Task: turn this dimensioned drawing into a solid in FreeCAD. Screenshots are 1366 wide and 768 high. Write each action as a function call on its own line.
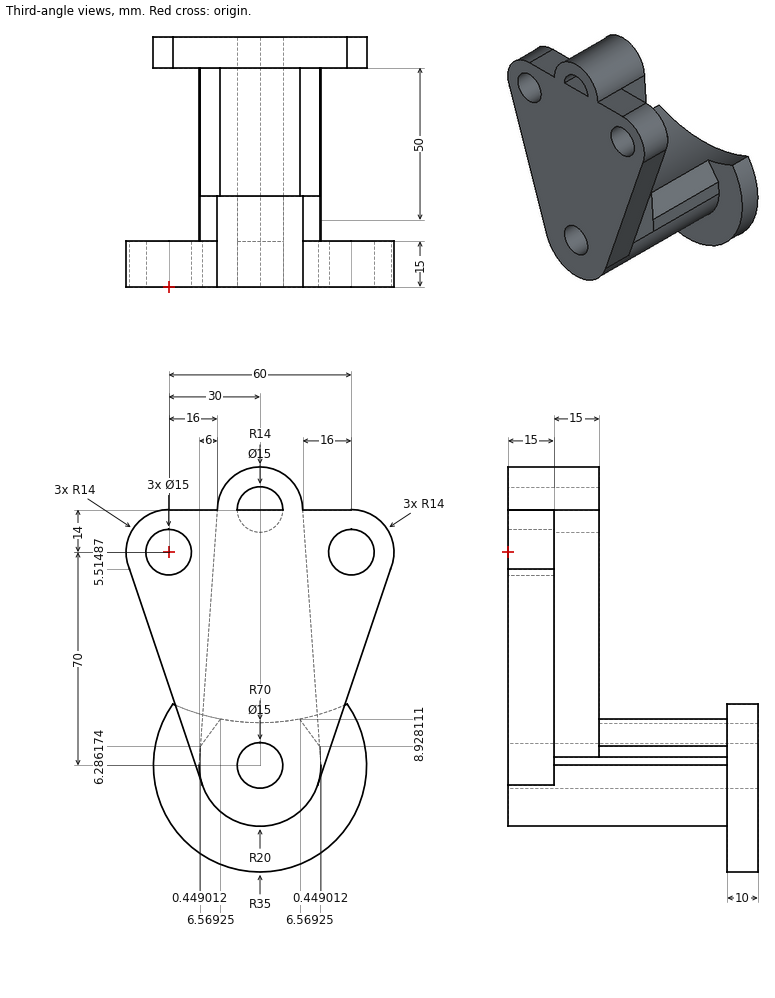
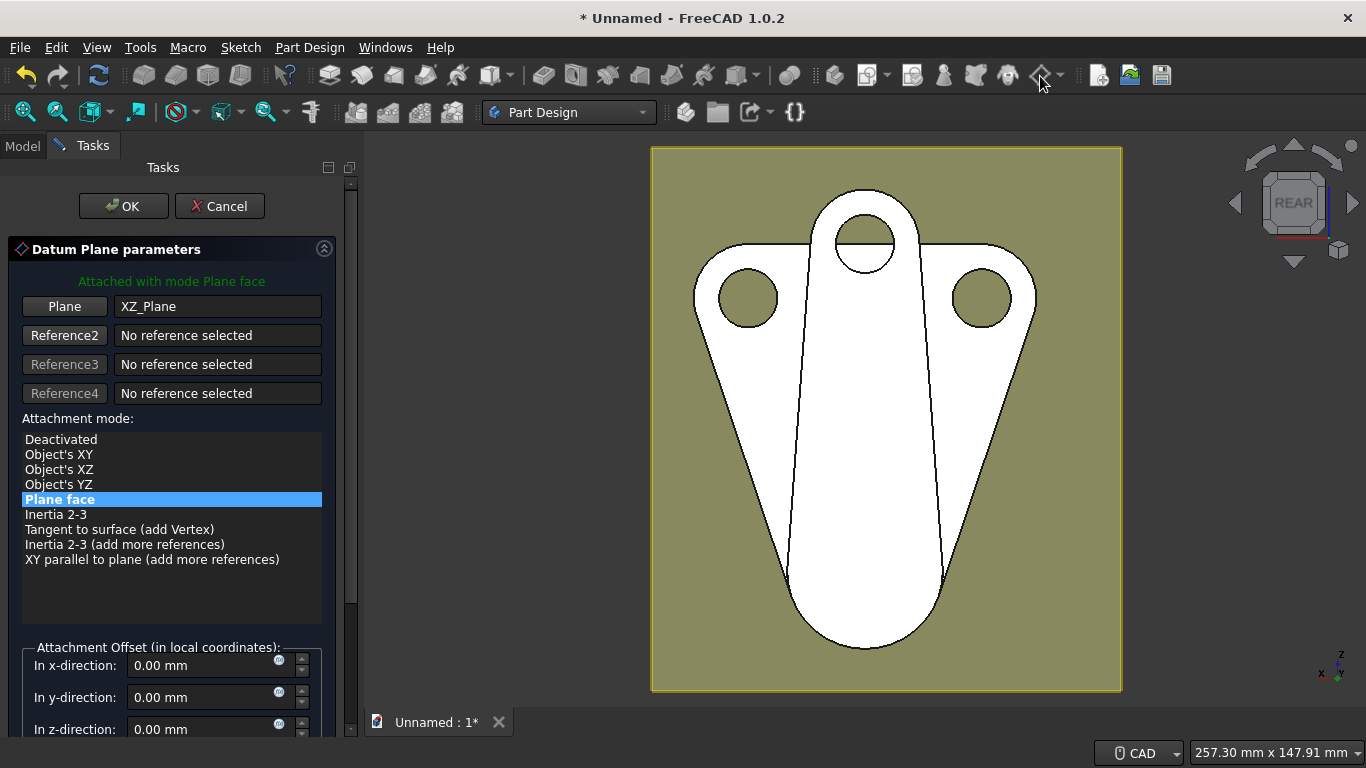
scroll(351, 456, down, 2)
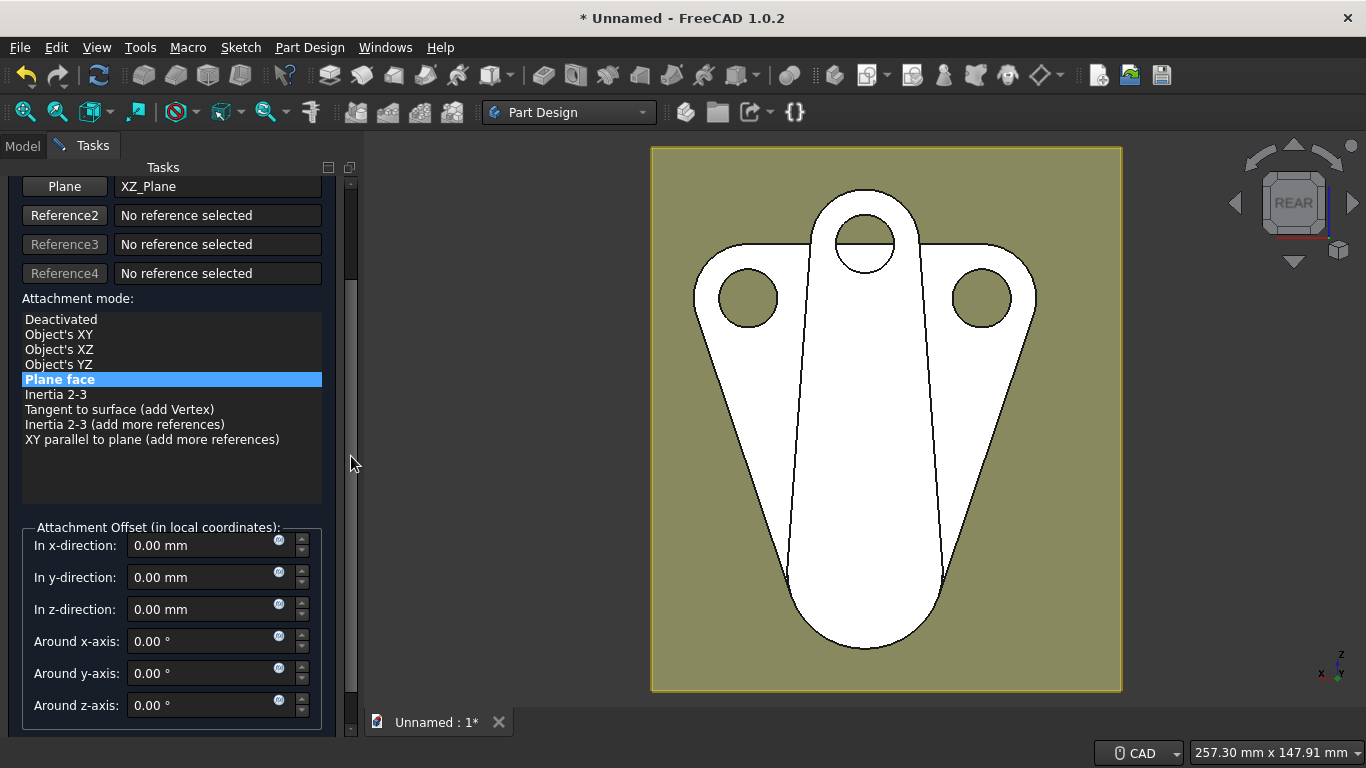
triple_click(210, 609)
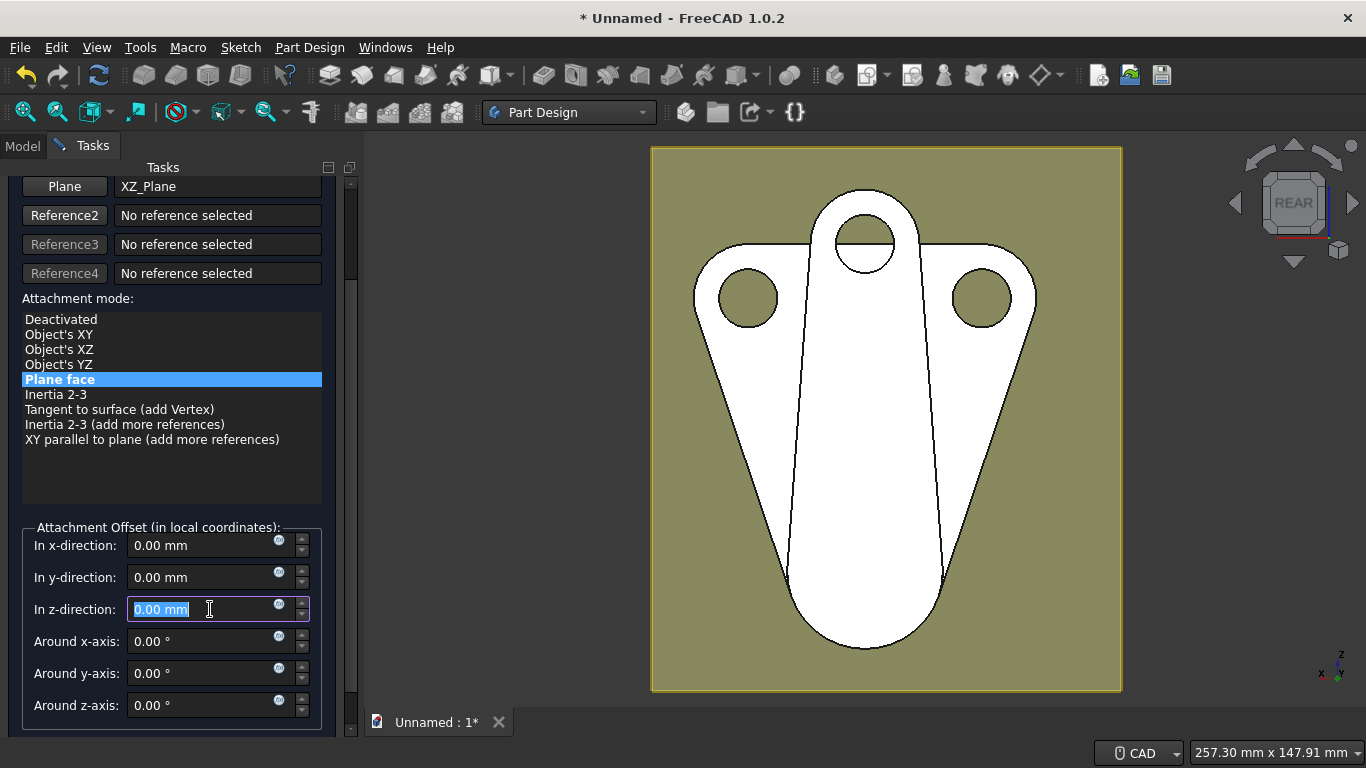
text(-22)
key(Tab)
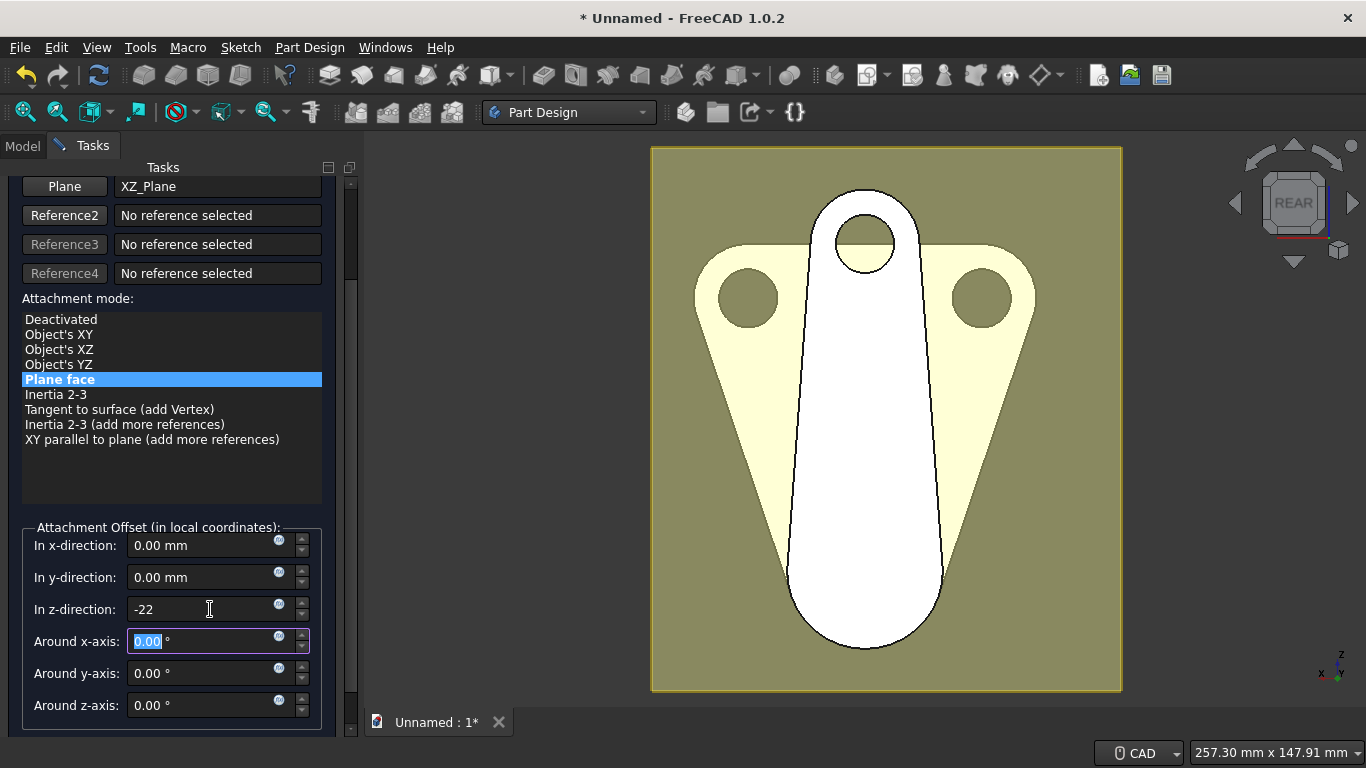
scroll(351, 456, up, 3)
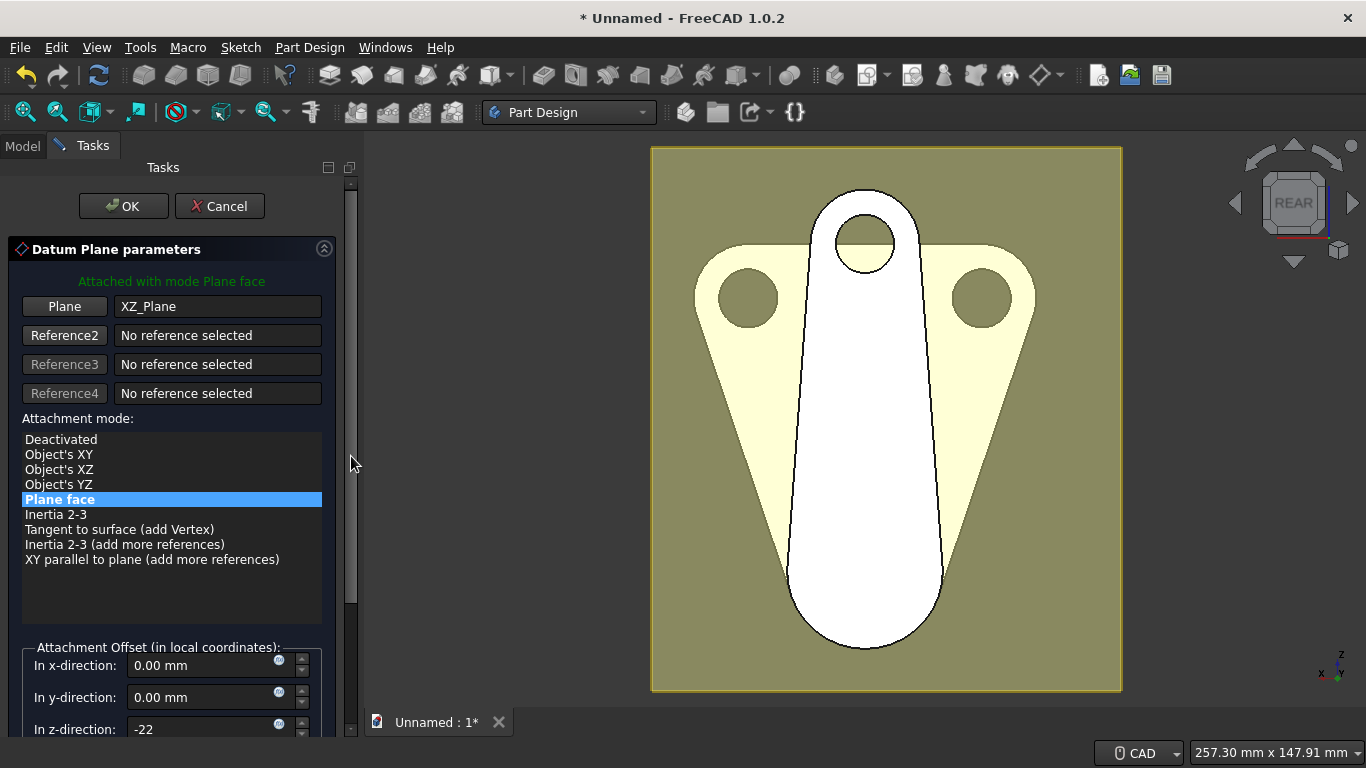
click(124, 206)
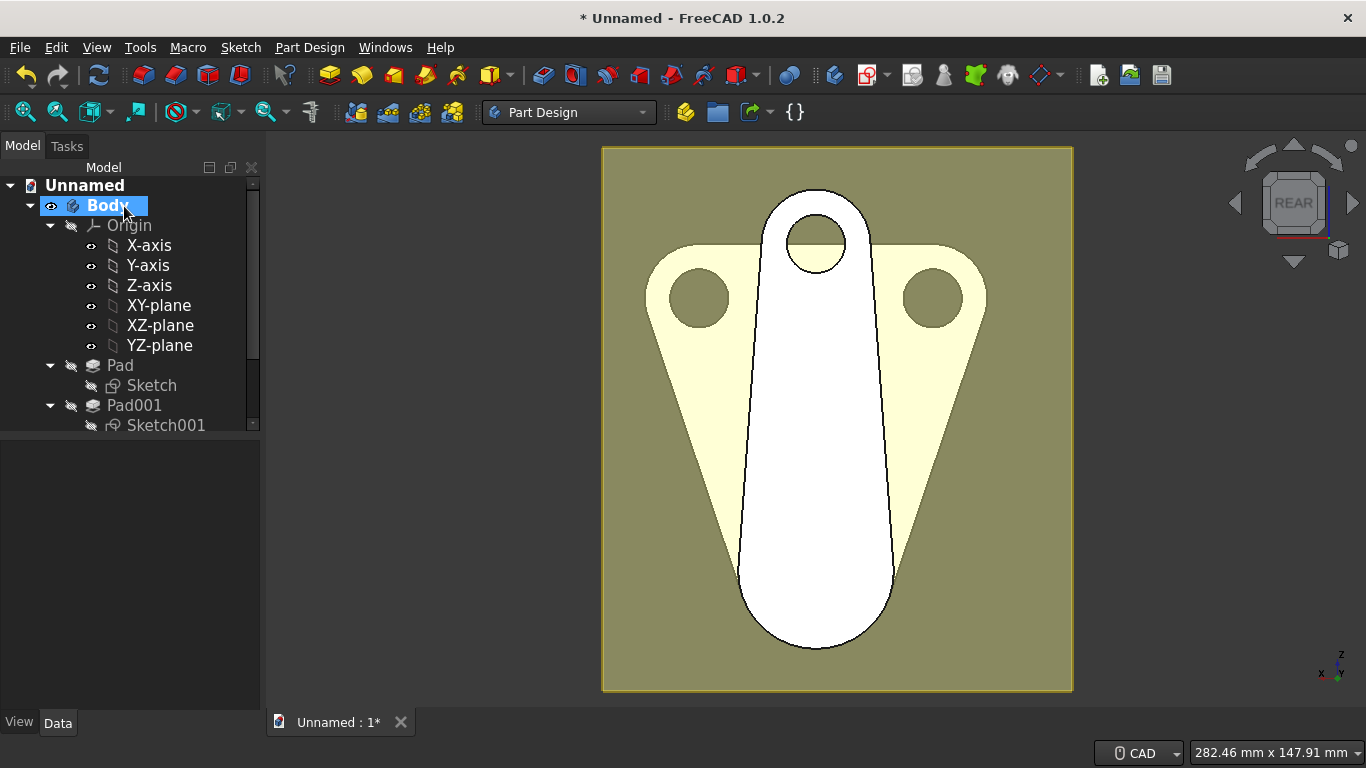
scroll(100, 301, down, 3)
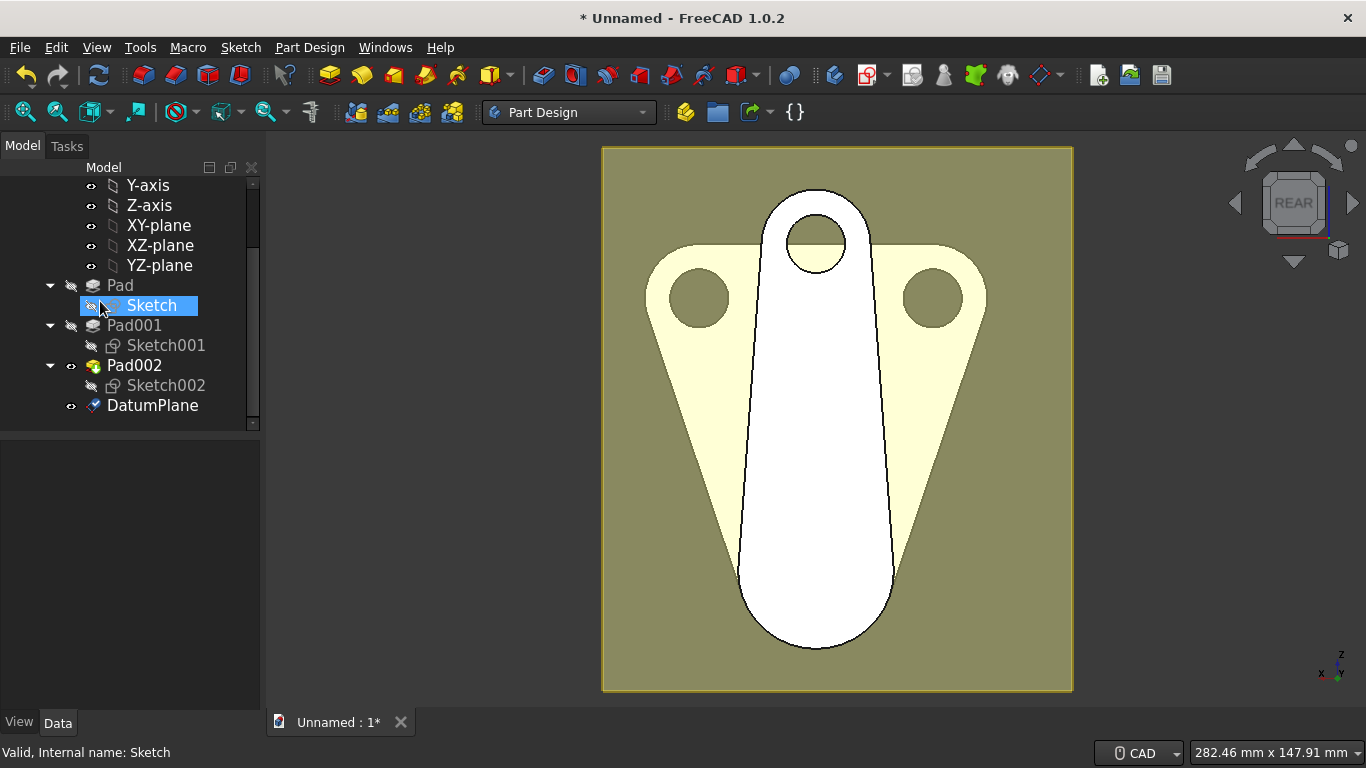
click(116, 406)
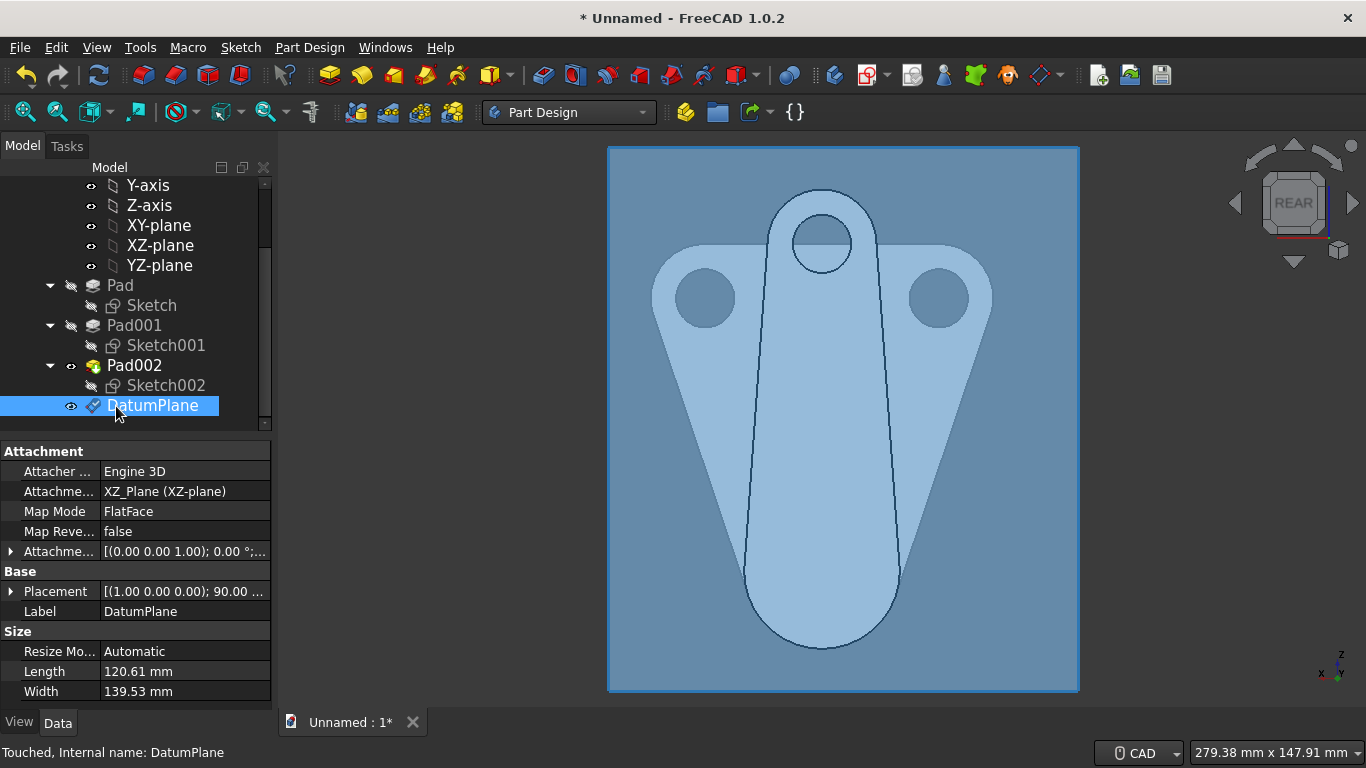
click(868, 76)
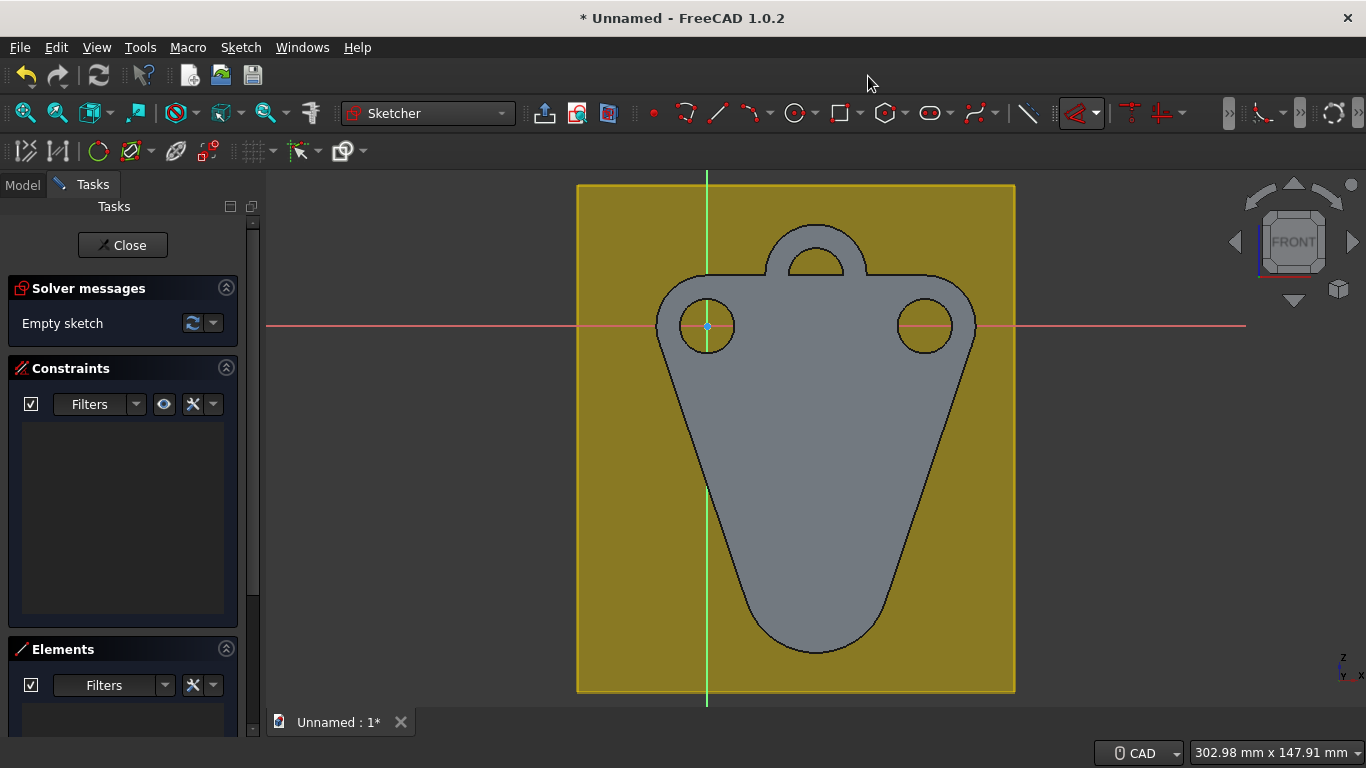
click(610, 114)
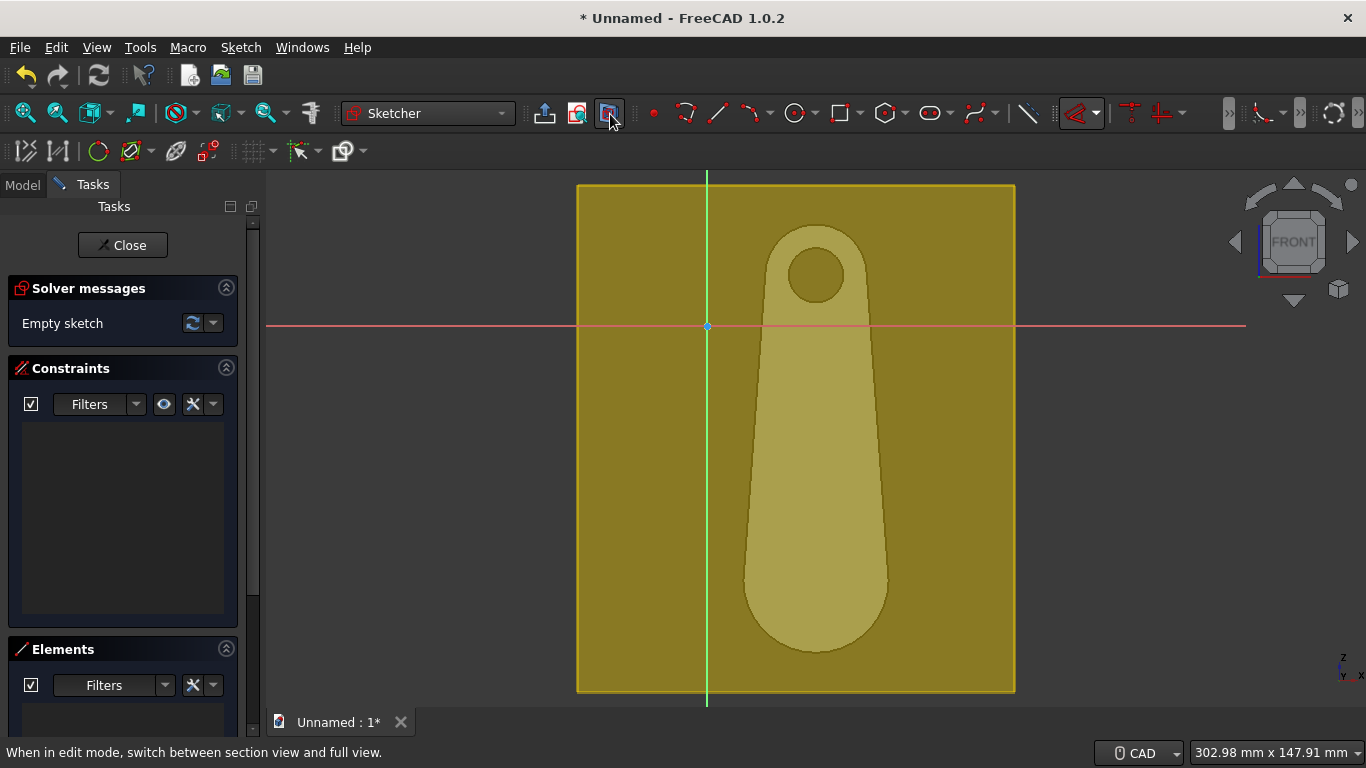
click(686, 114)